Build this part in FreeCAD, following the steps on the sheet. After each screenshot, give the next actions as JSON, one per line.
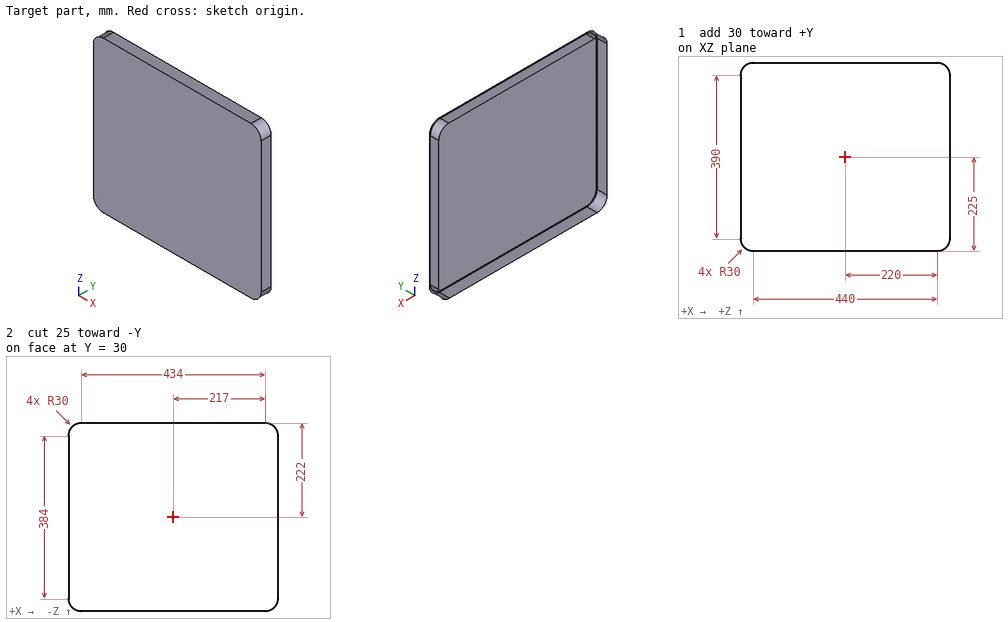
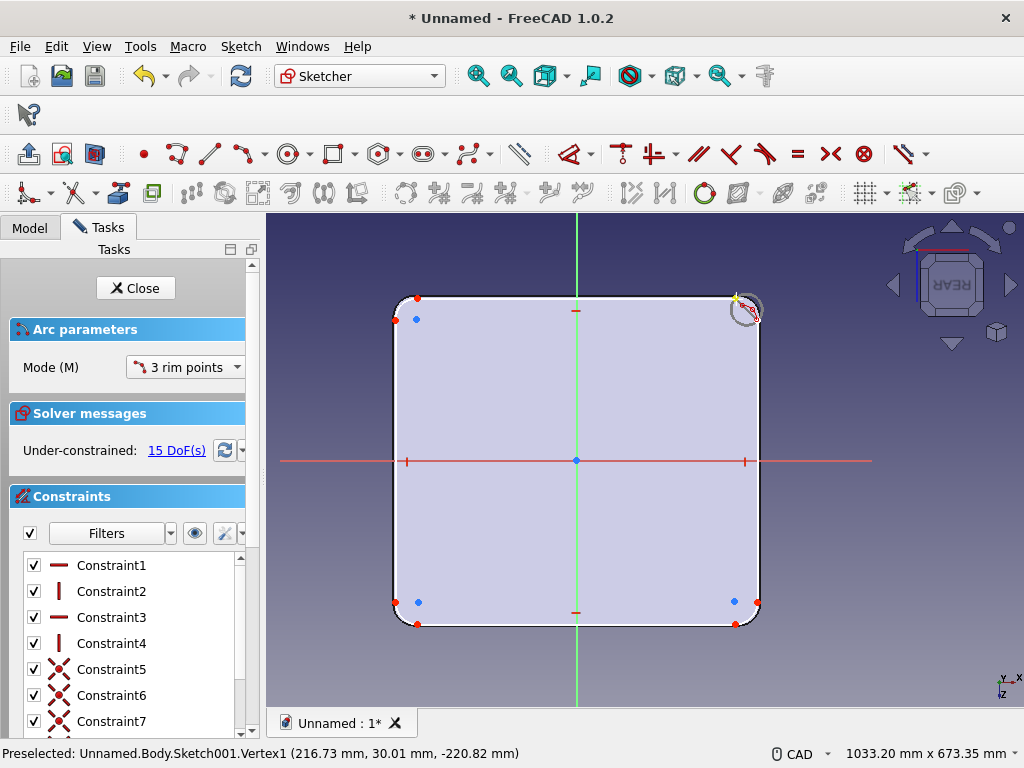
{"action": "scroll", "coordinate": [751, 304], "scroll_direction": "up", "scroll_amount": 5}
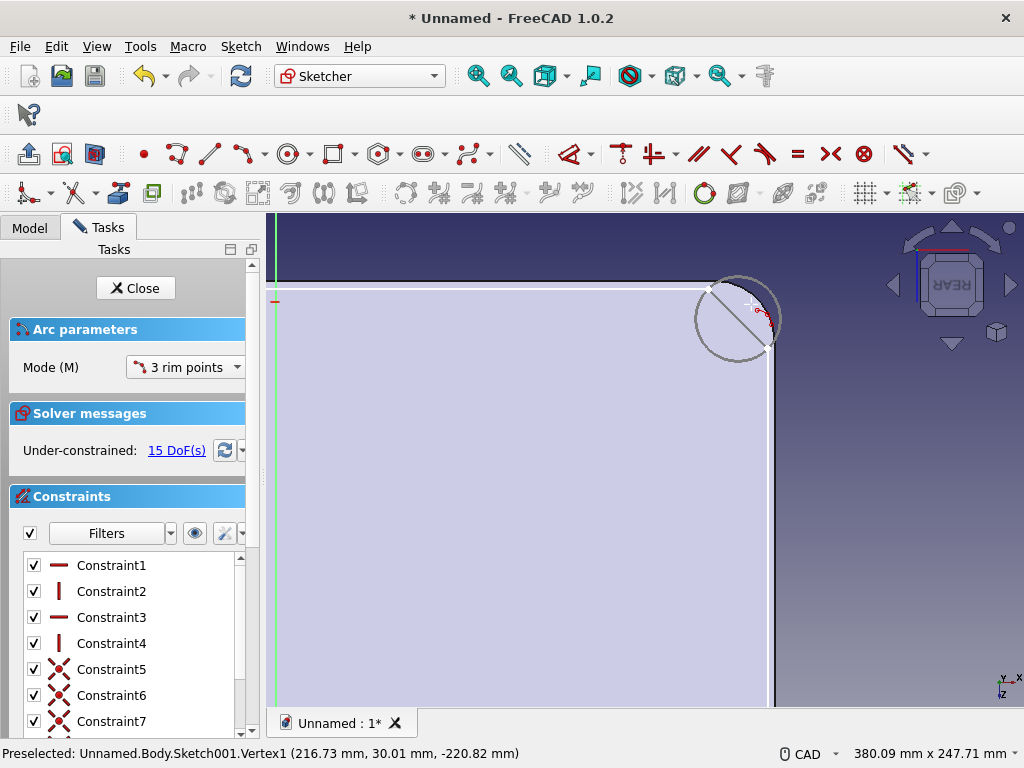
{"action": "left_click", "coordinate": [751, 304]}
{"action": "key", "text": "Escape"}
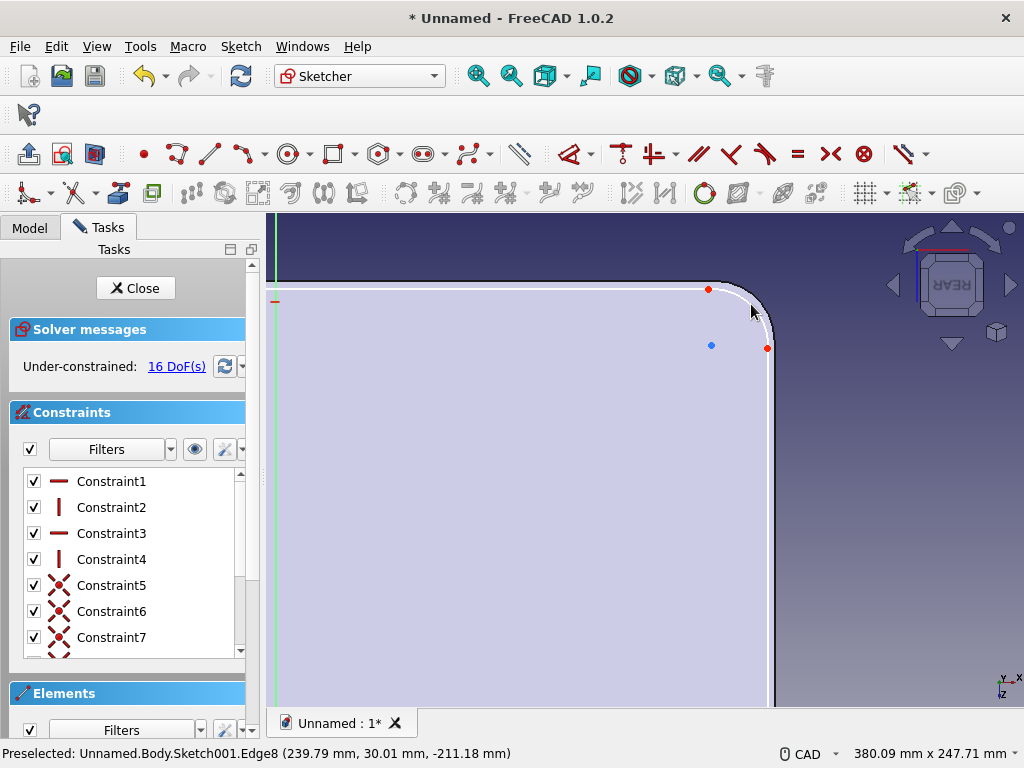
{"action": "left_click", "coordinate": [449, 289]}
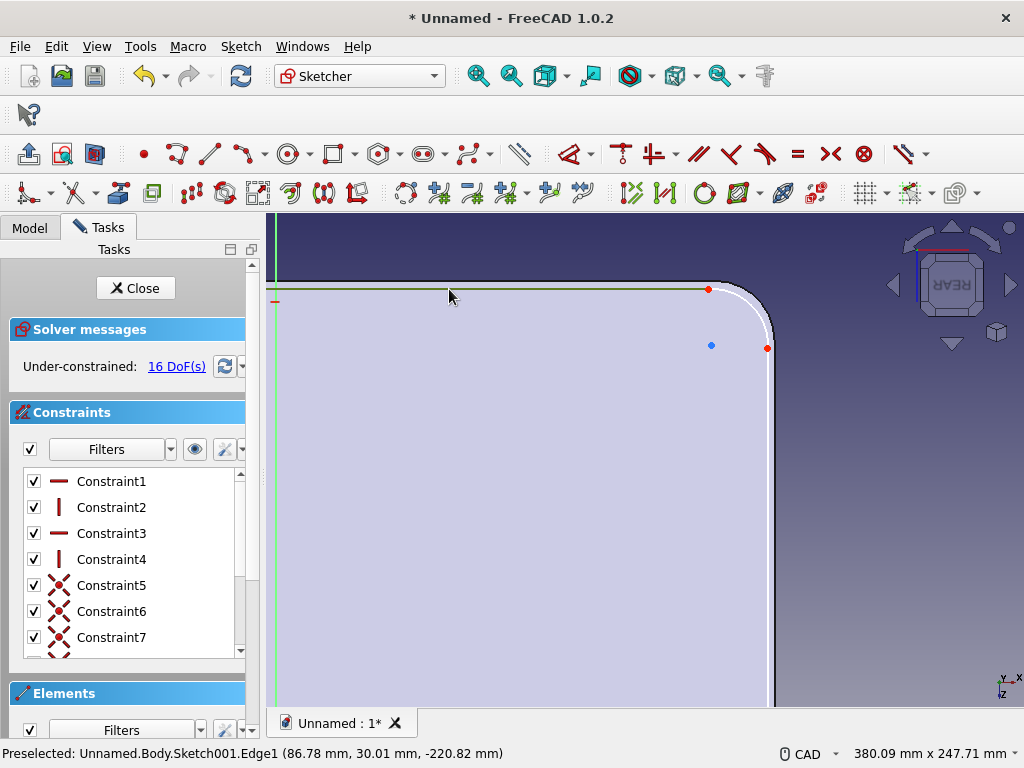
{"action": "scroll", "coordinate": [751, 303], "scroll_direction": "down", "scroll_amount": 5}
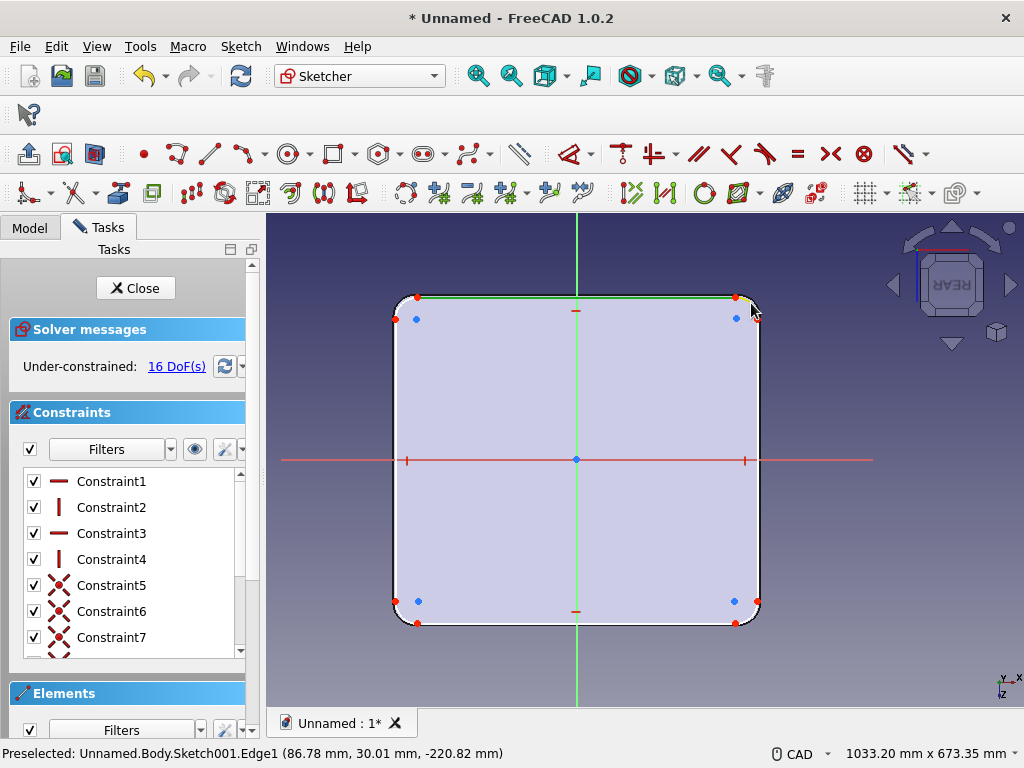
{"action": "scroll", "coordinate": [407, 300], "scroll_direction": "up", "scroll_amount": 2}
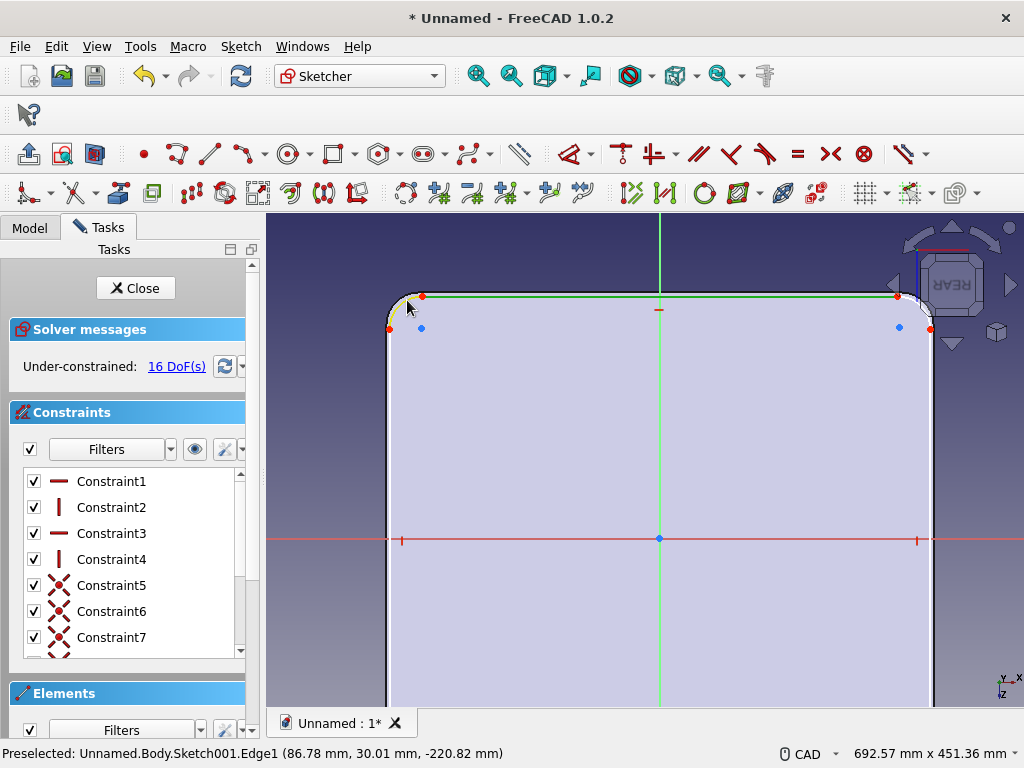
{"action": "left_click", "coordinate": [408, 300]}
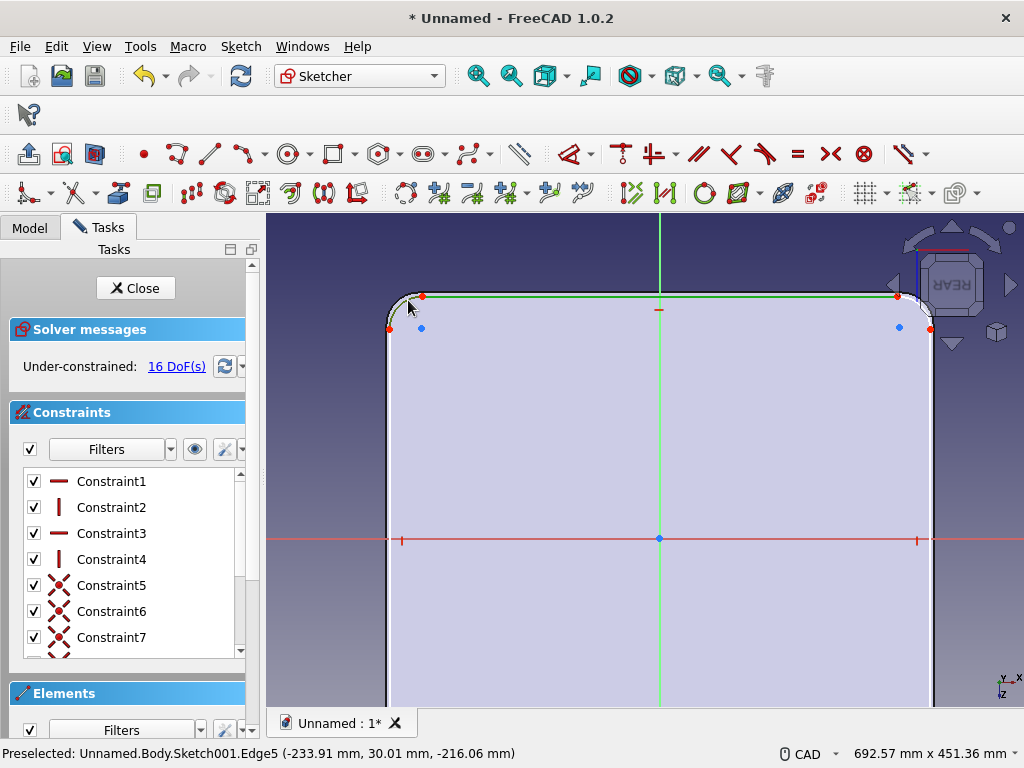
{"action": "left_click", "coordinate": [765, 154]}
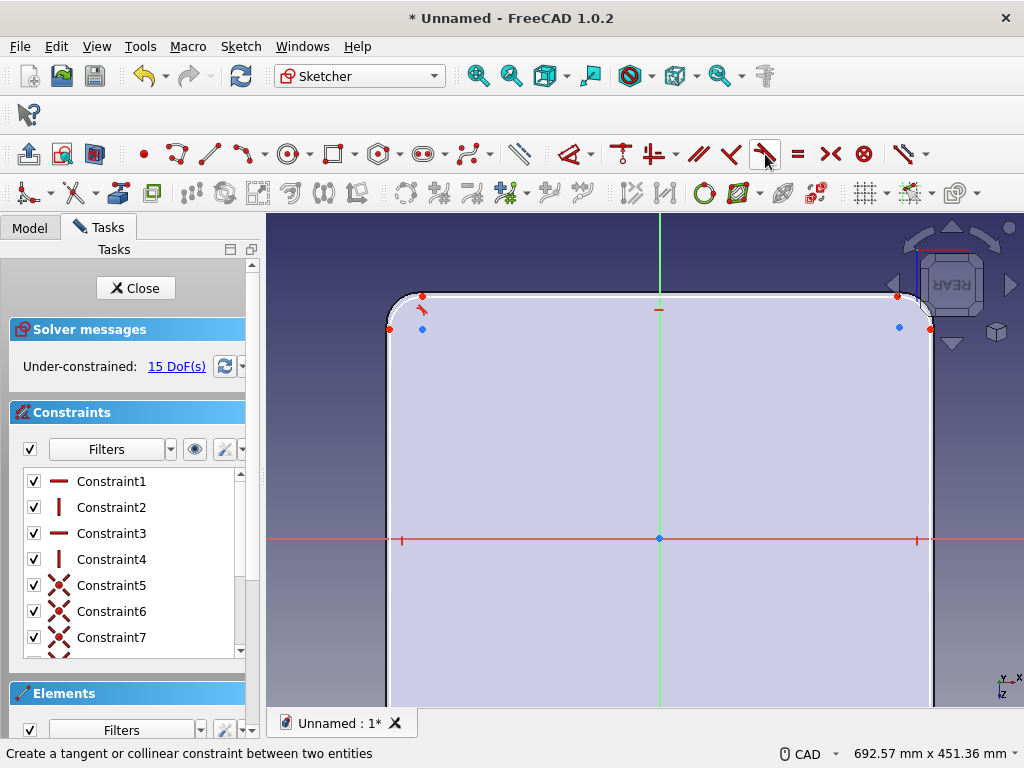
{"action": "left_click", "coordinate": [755, 297]}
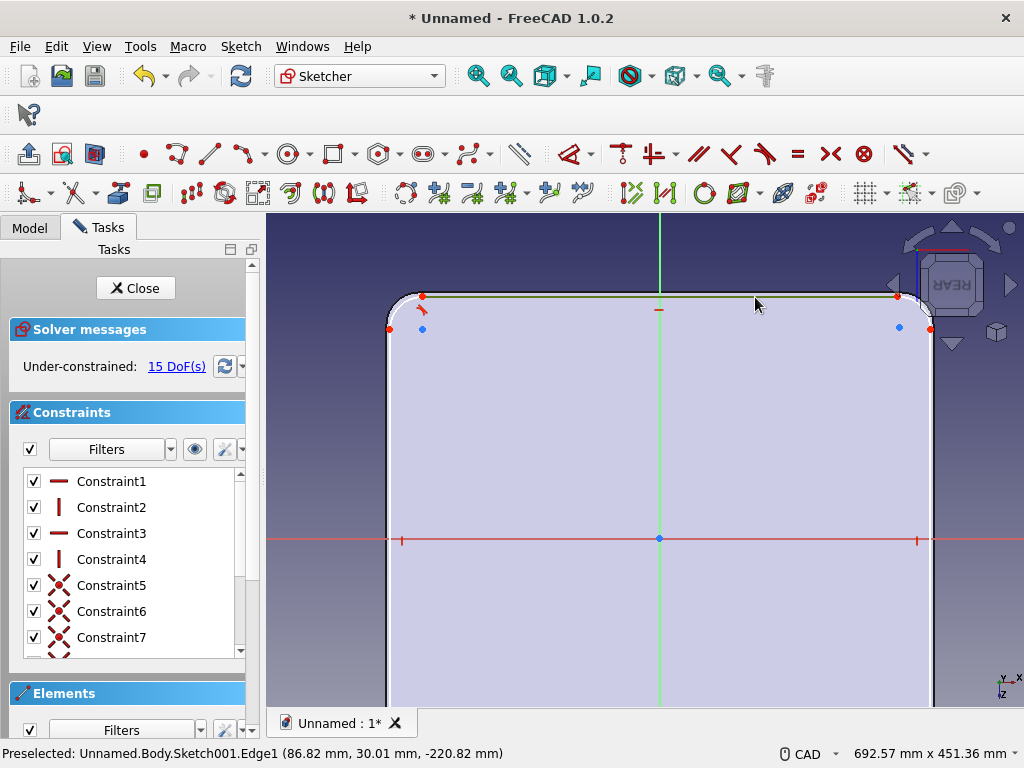
{"action": "scroll", "coordinate": [407, 300], "scroll_direction": "down", "scroll_amount": 2}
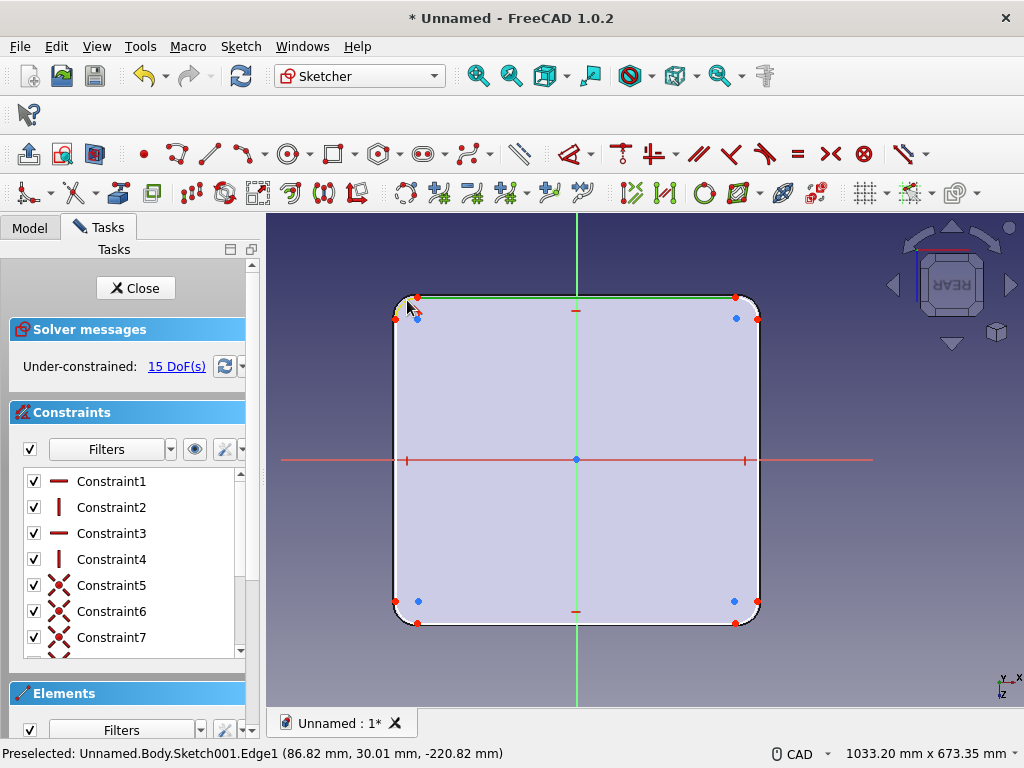
{"action": "scroll", "coordinate": [756, 310], "scroll_direction": "up", "scroll_amount": 2}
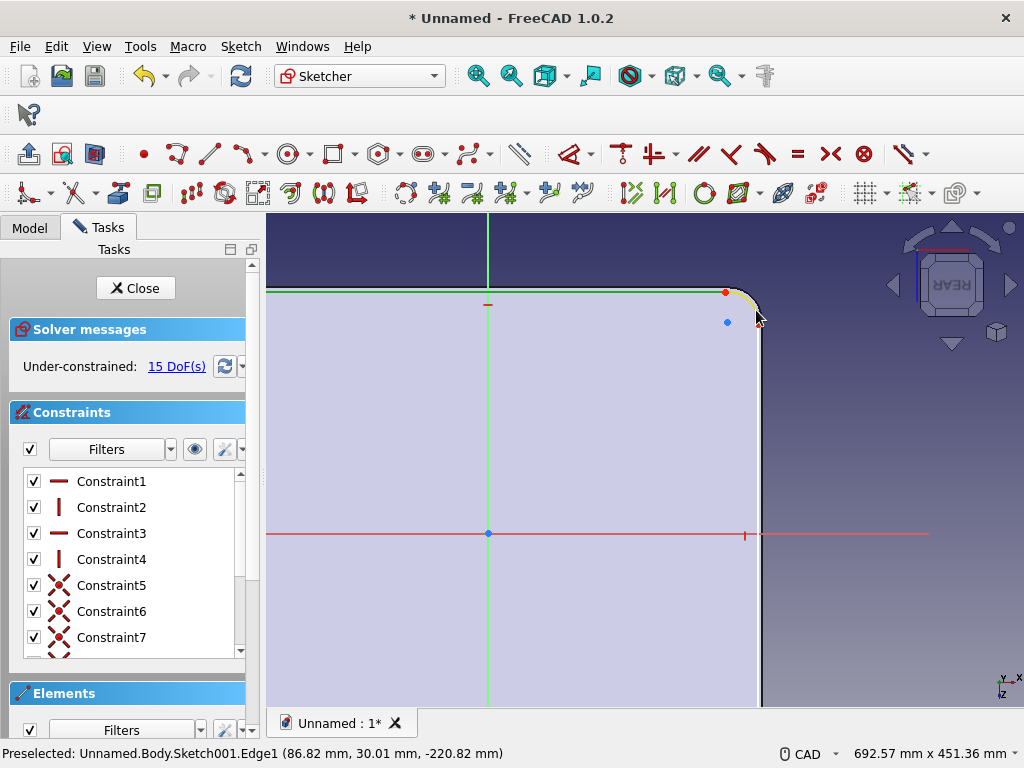
{"action": "left_click", "coordinate": [755, 310]}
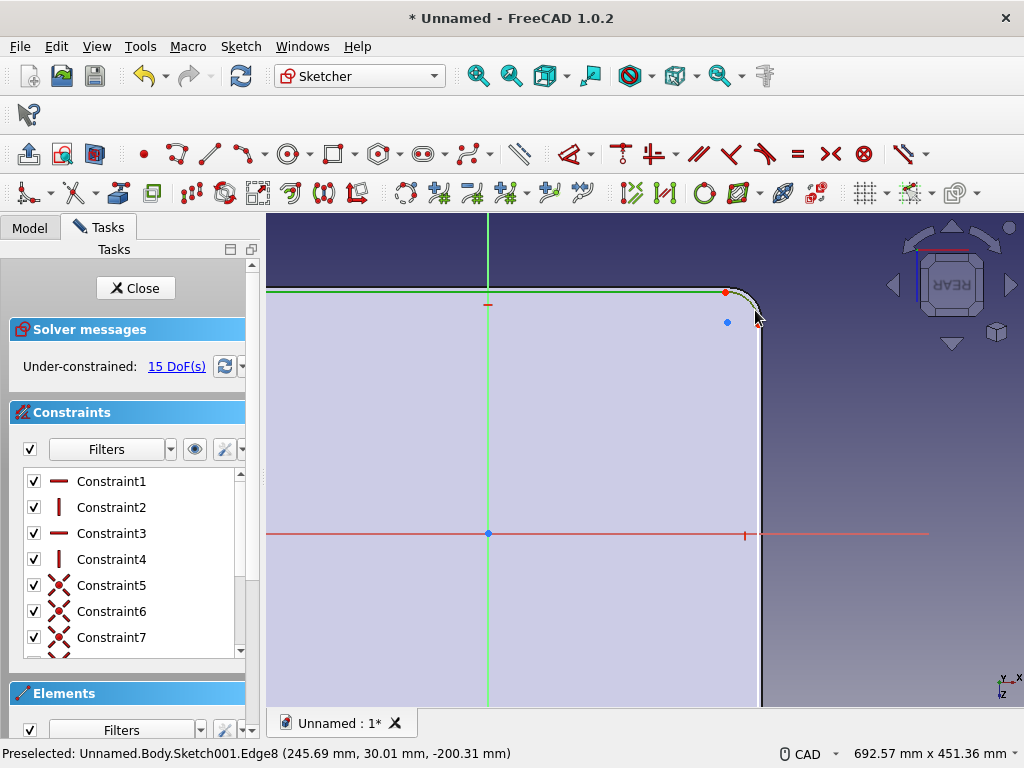
{"action": "left_click", "coordinate": [765, 154]}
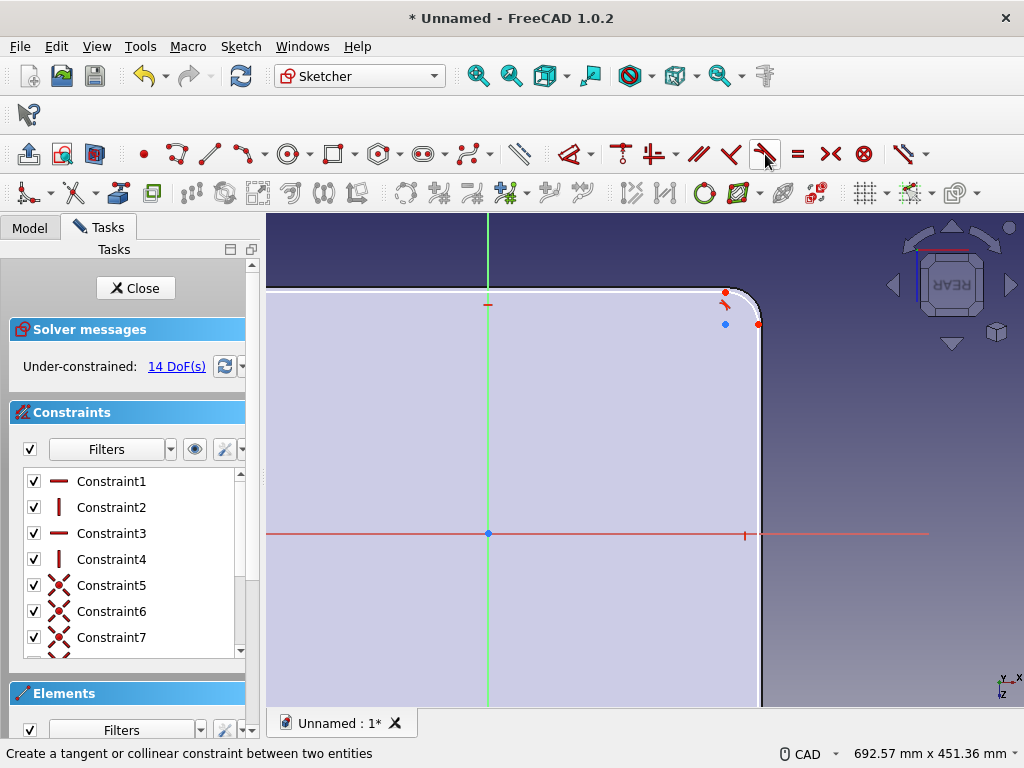
{"action": "scroll", "coordinate": [756, 310], "scroll_direction": "down", "scroll_amount": 2}